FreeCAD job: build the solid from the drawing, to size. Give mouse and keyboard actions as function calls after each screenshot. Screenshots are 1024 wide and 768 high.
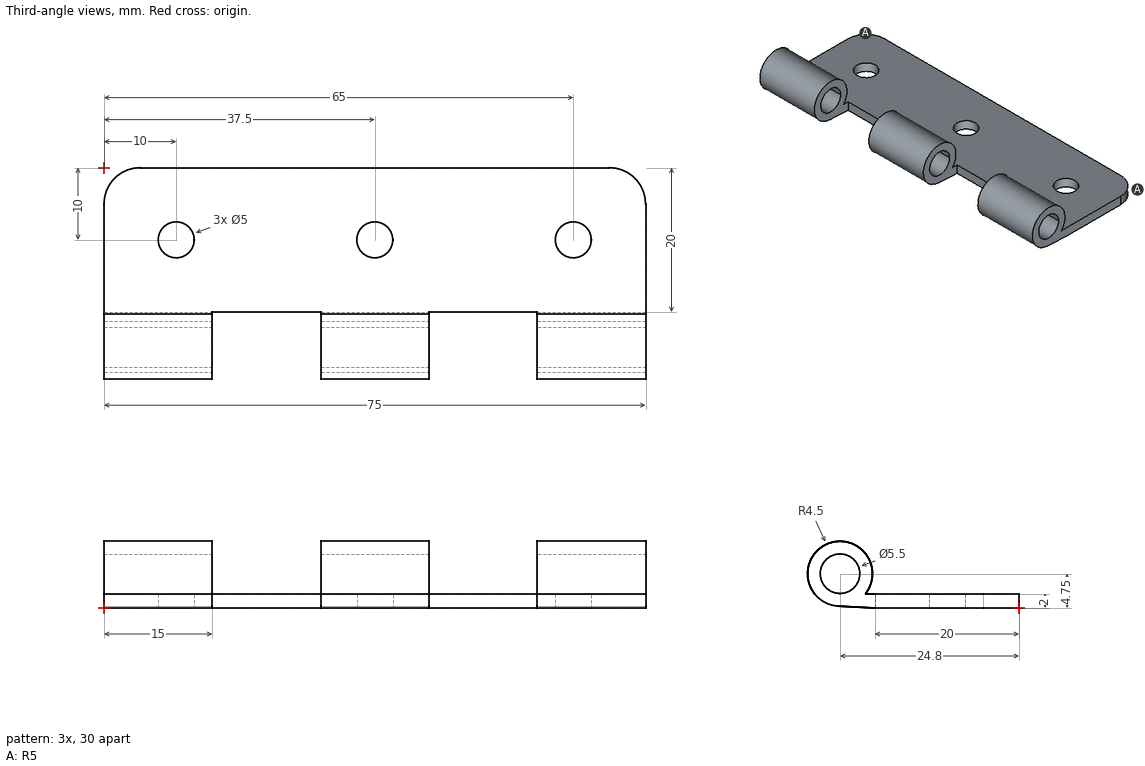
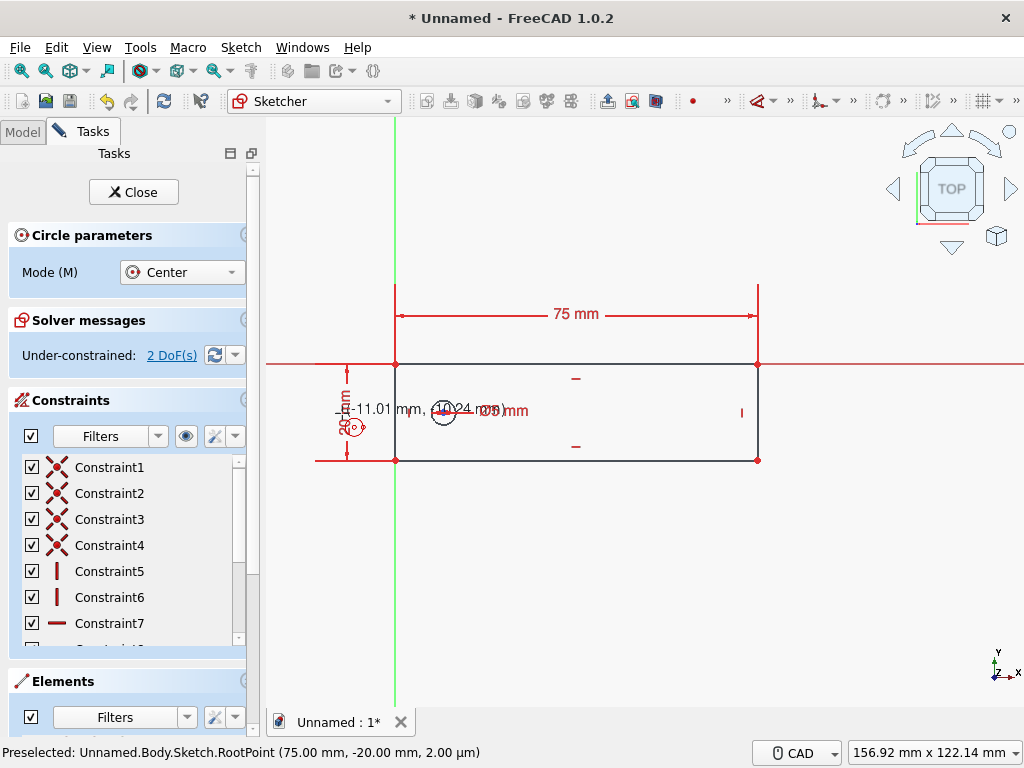
scroll(576, 413, up, 4)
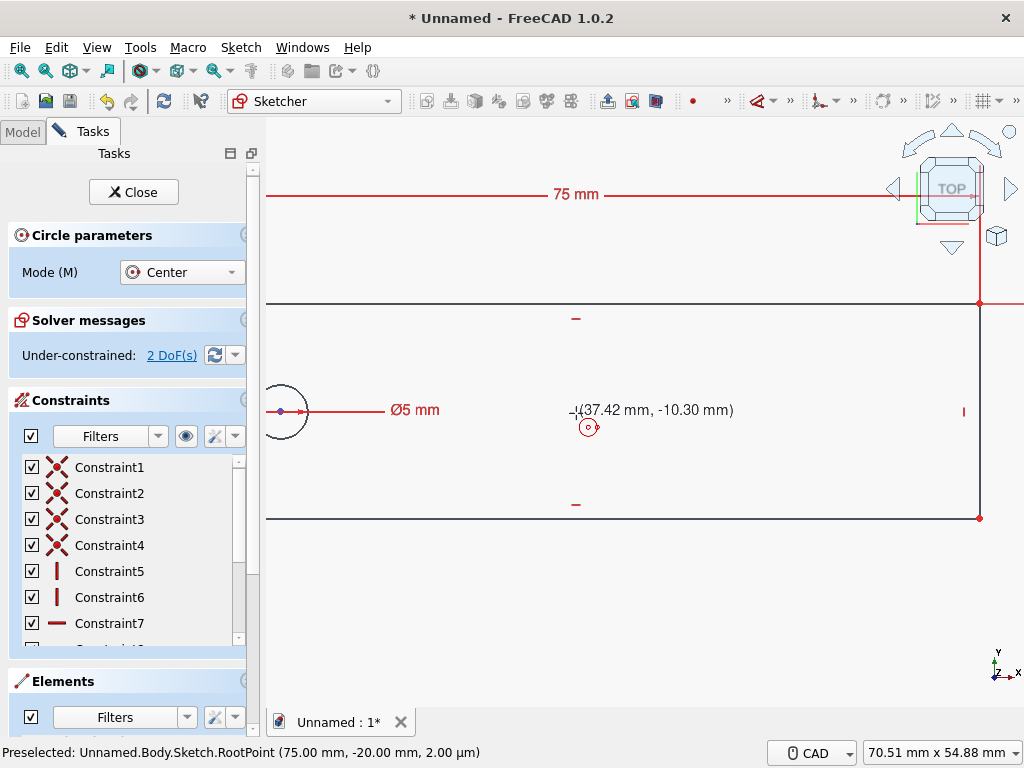
click(576, 411)
move(595, 392)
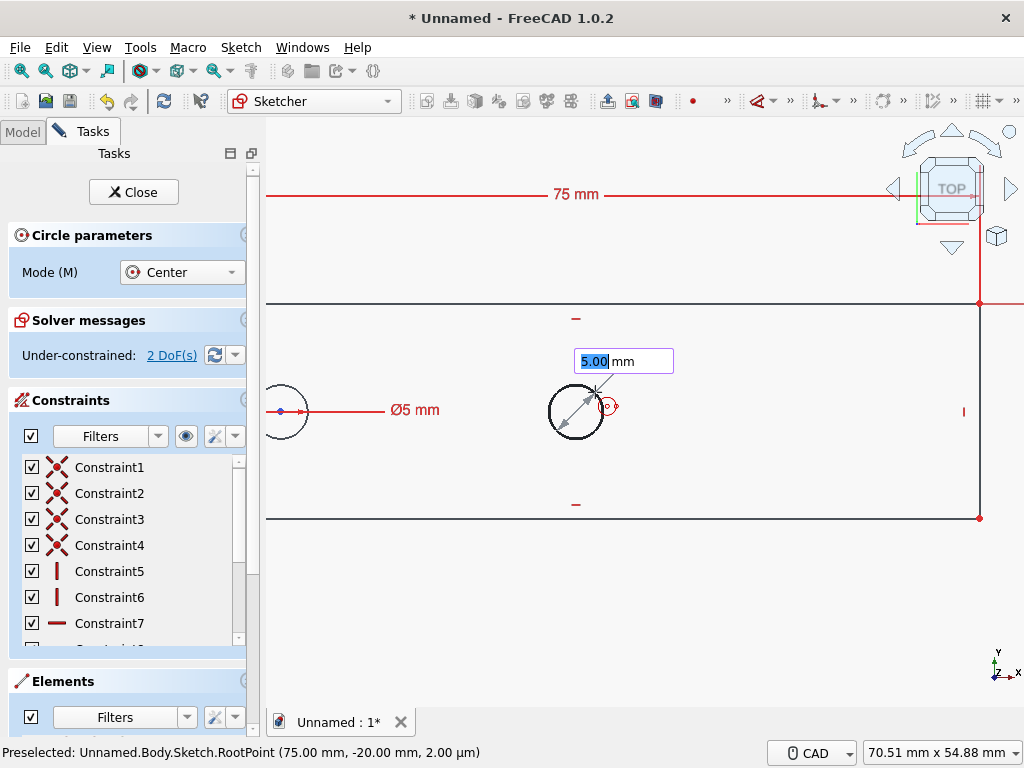
text(5)
key(Return)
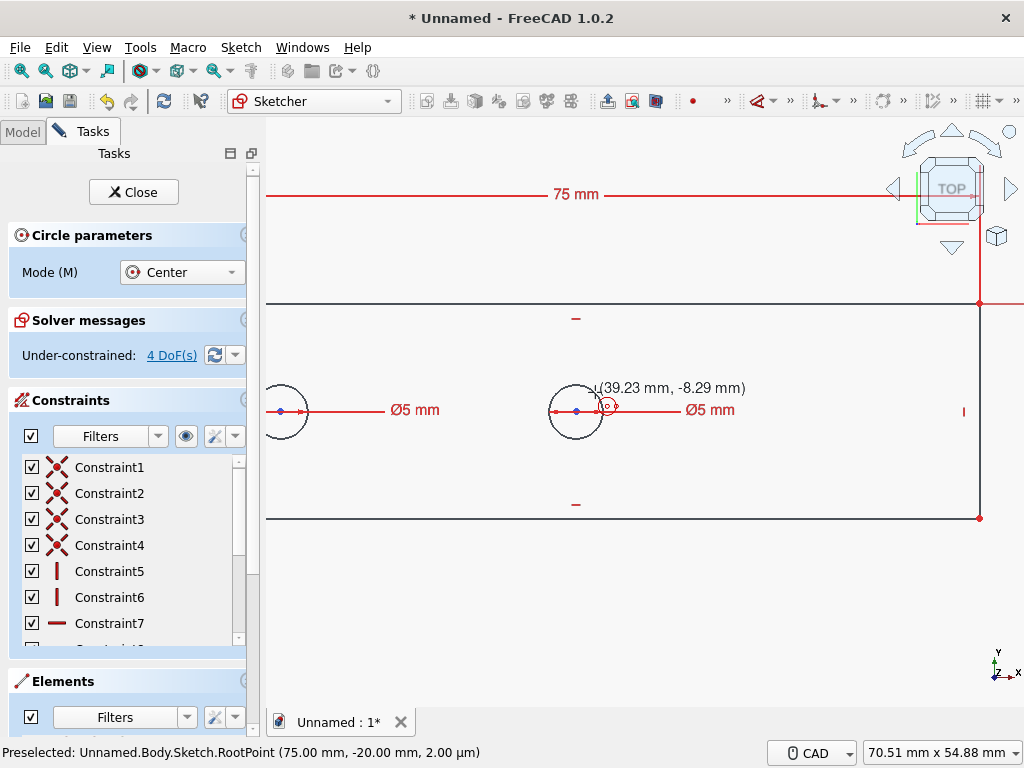
scroll(577, 413, down, 4)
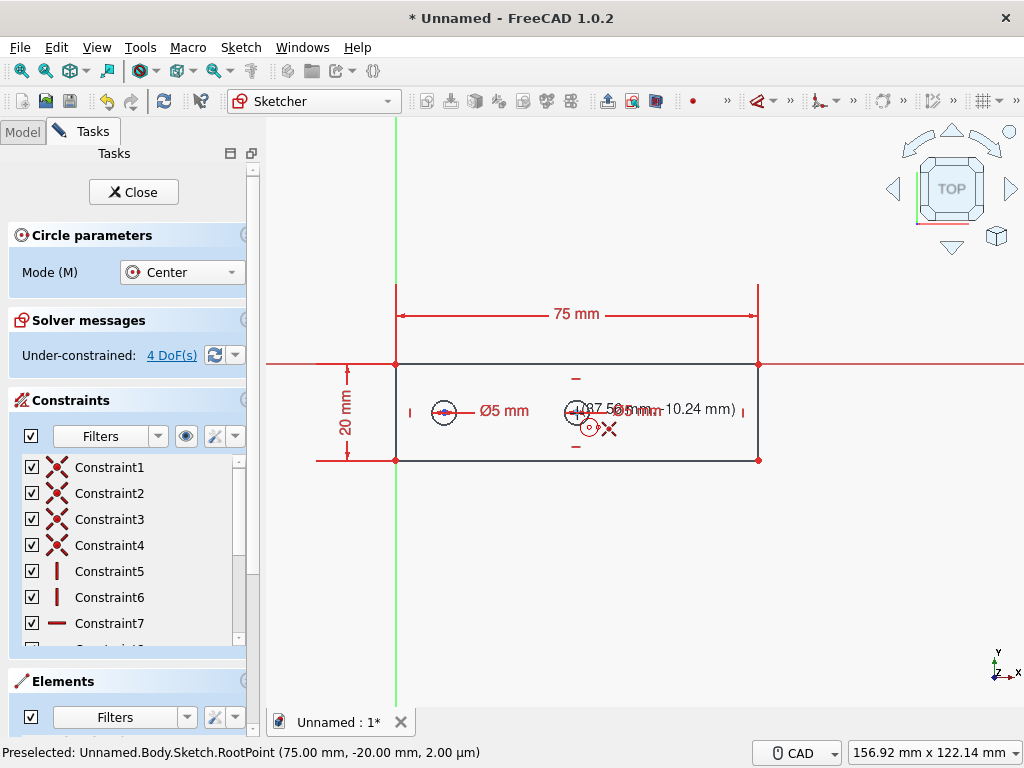
scroll(710, 413, up, 4)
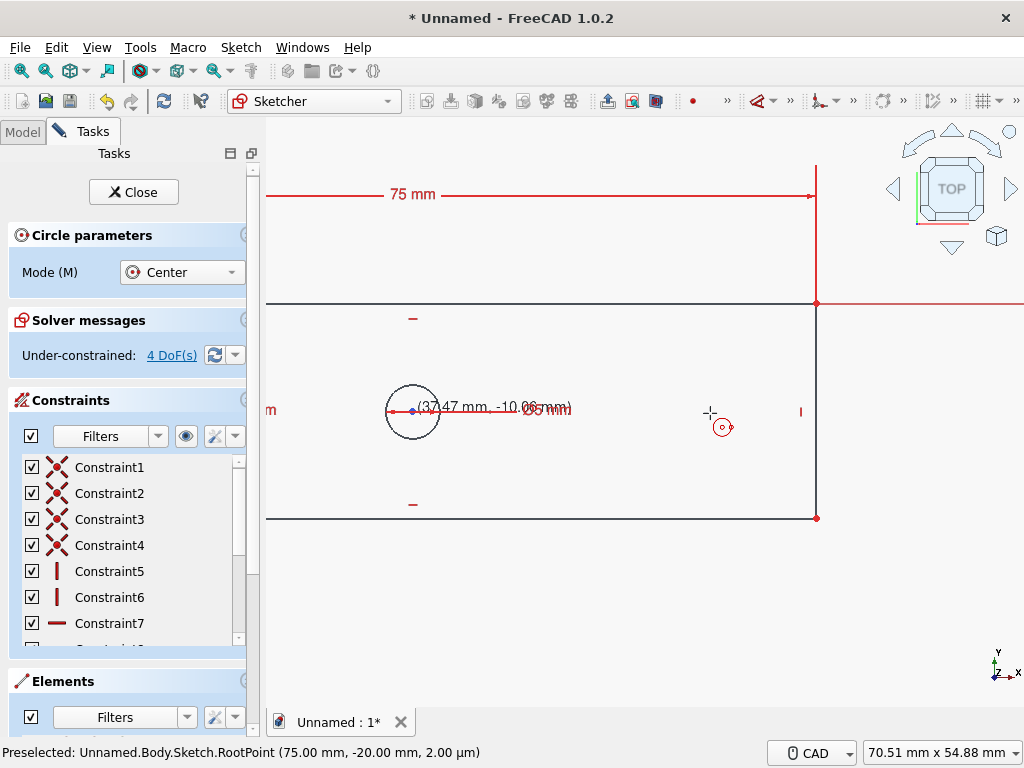
click(709, 411)
move(728, 392)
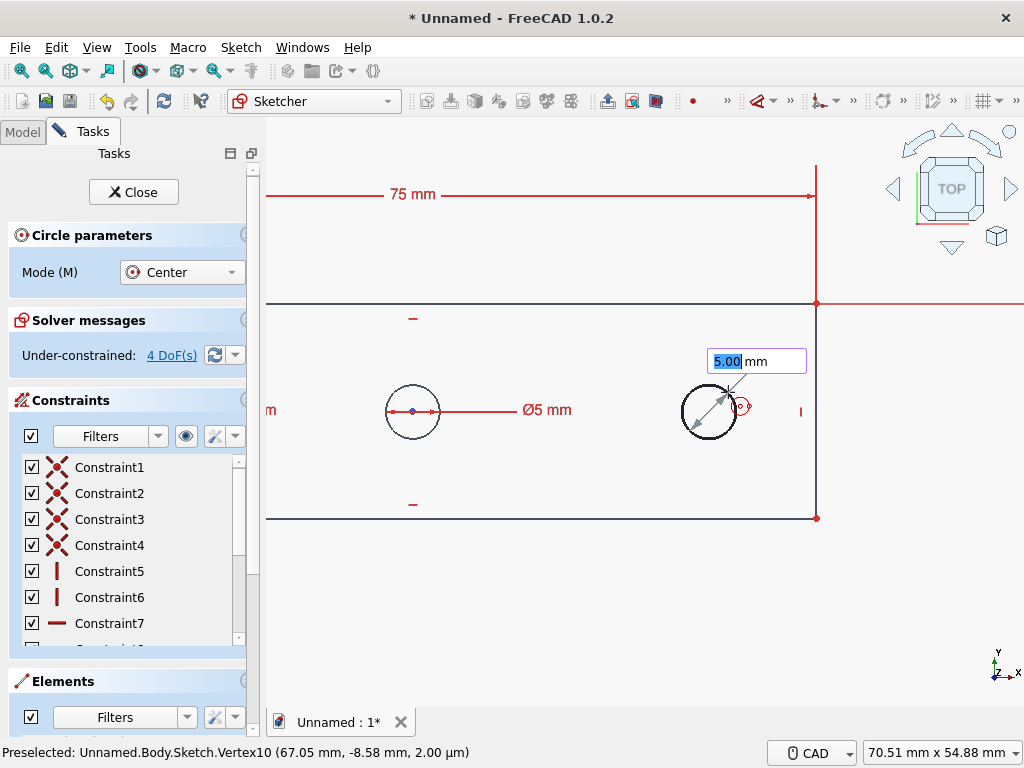
text(5)
key(Return)
key(Escape)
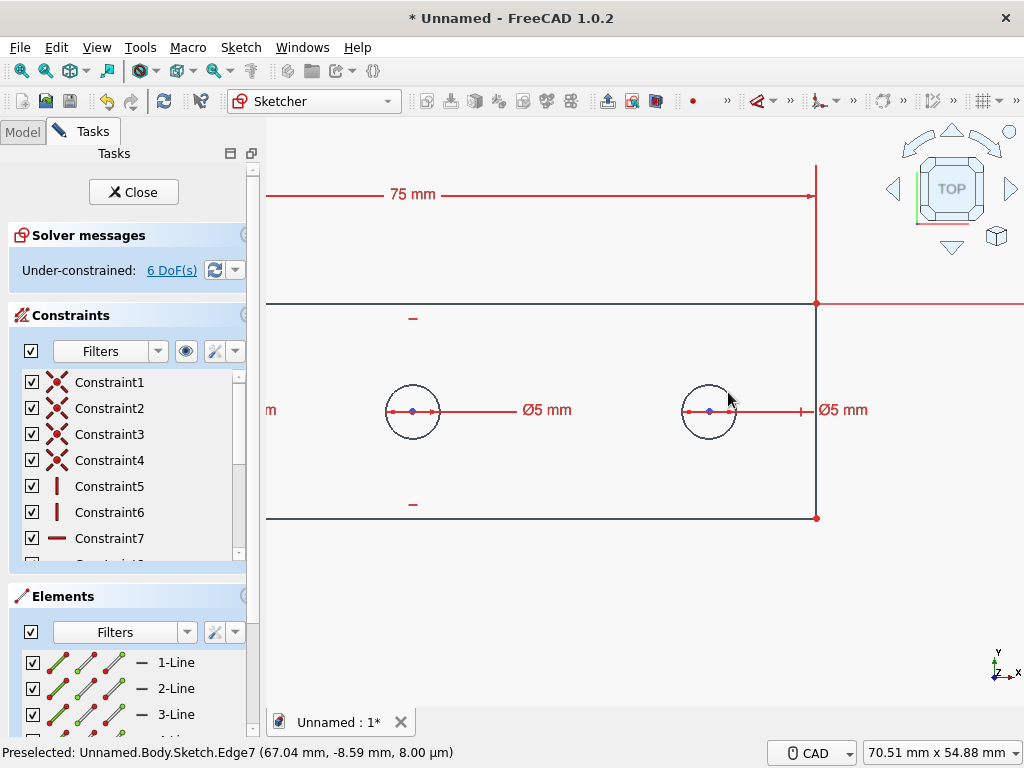
click(758, 102)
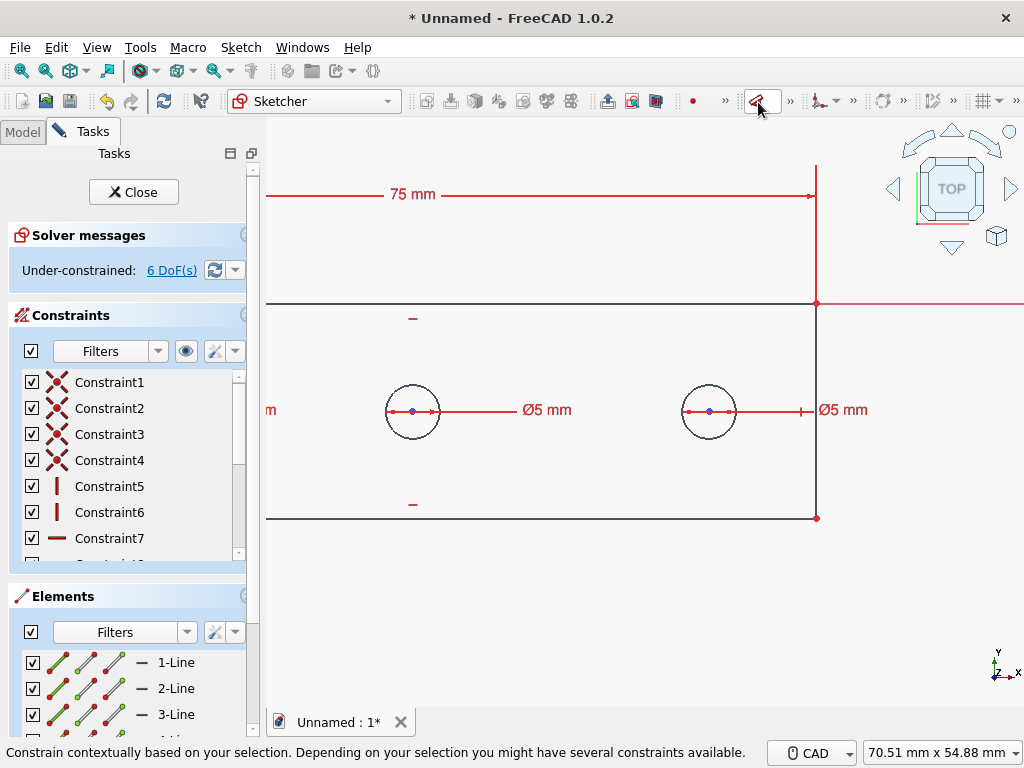
scroll(710, 413, down, 4)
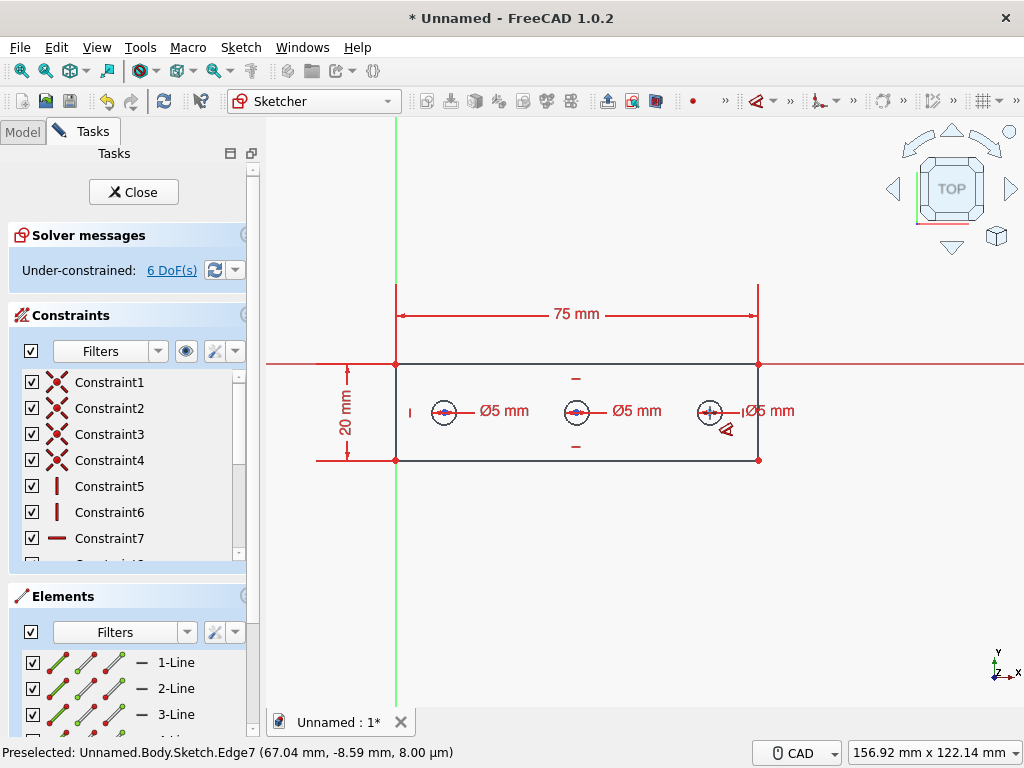
click(444, 413)
click(420, 330)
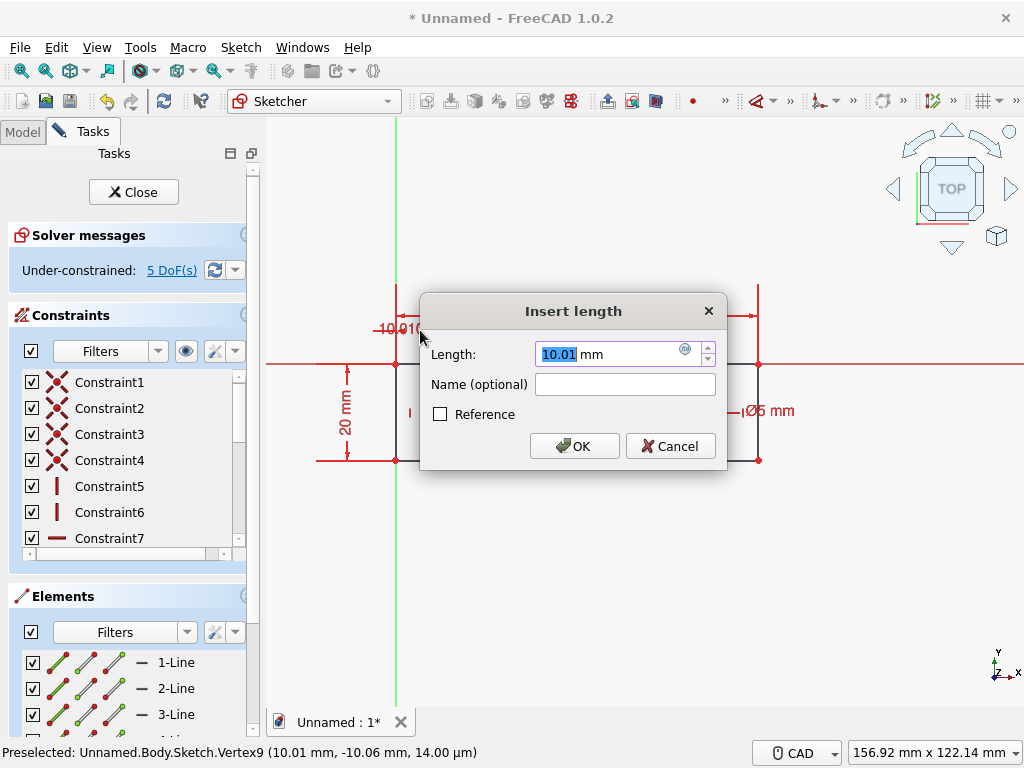
text(10)
key(Return)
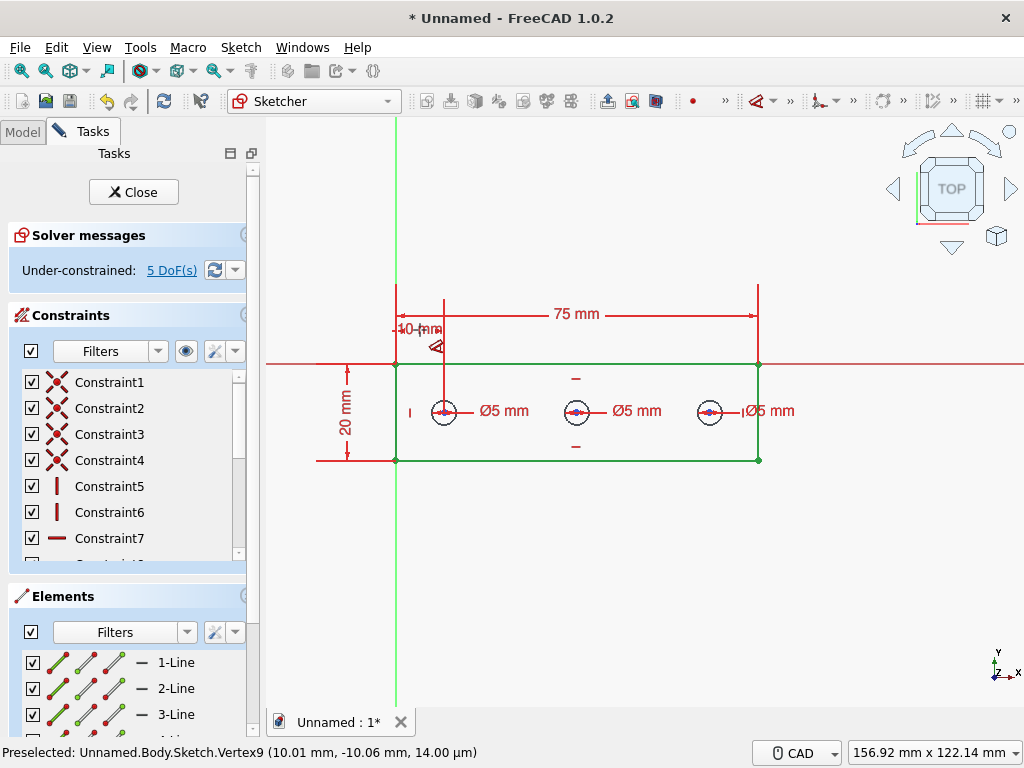
click(444, 413)
click(362, 389)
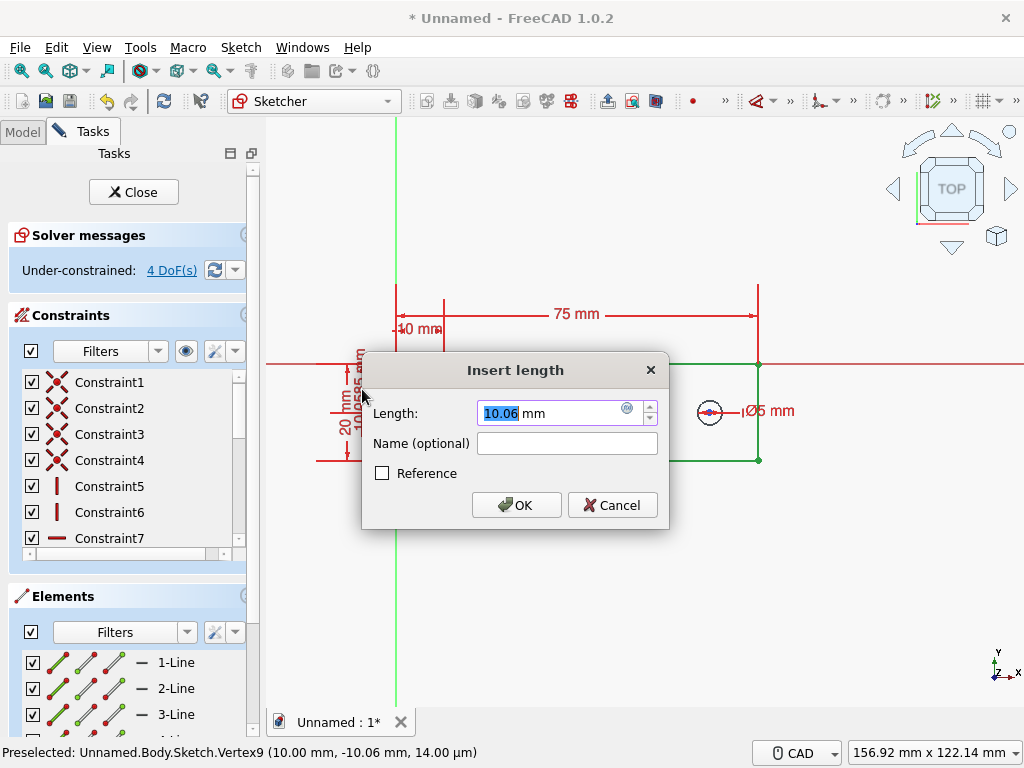
text(10)
key(Return)